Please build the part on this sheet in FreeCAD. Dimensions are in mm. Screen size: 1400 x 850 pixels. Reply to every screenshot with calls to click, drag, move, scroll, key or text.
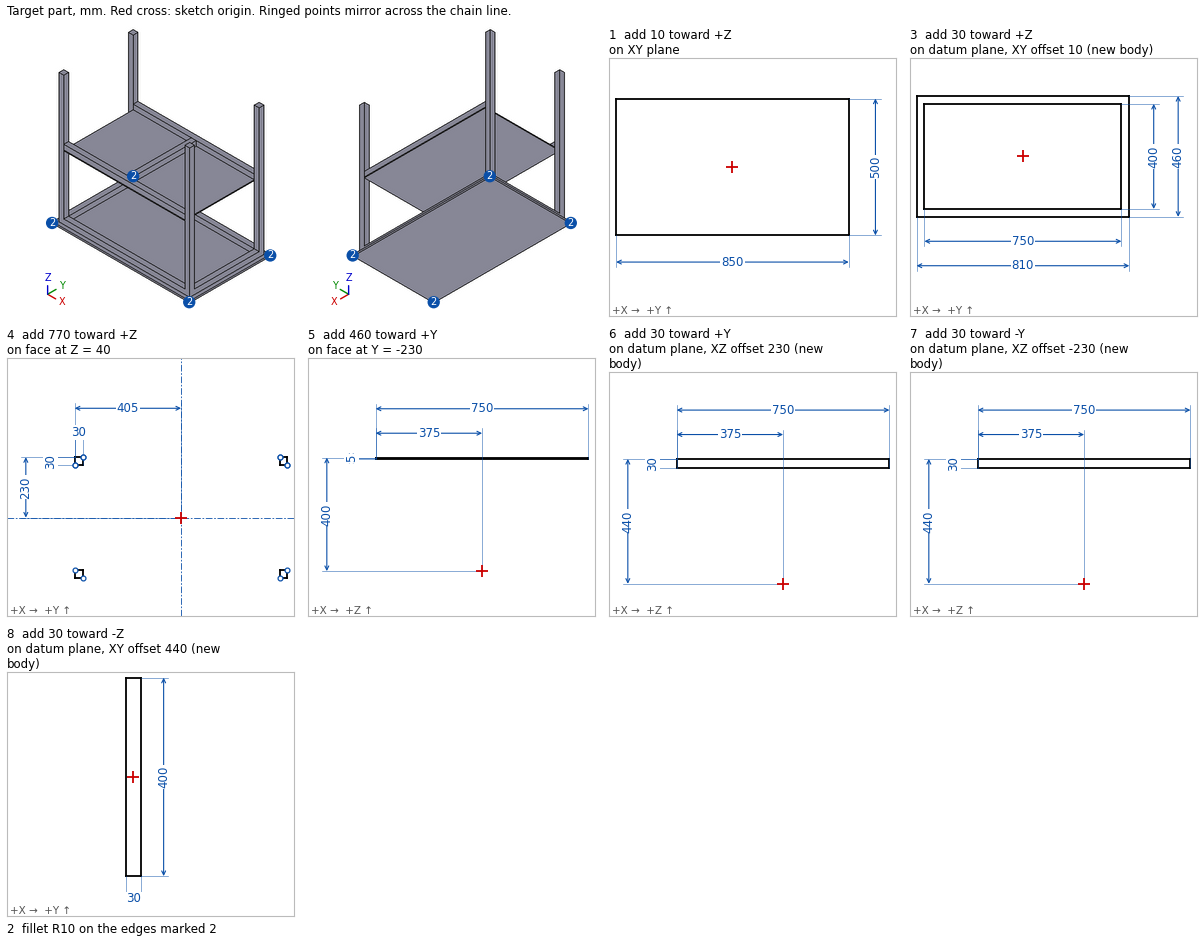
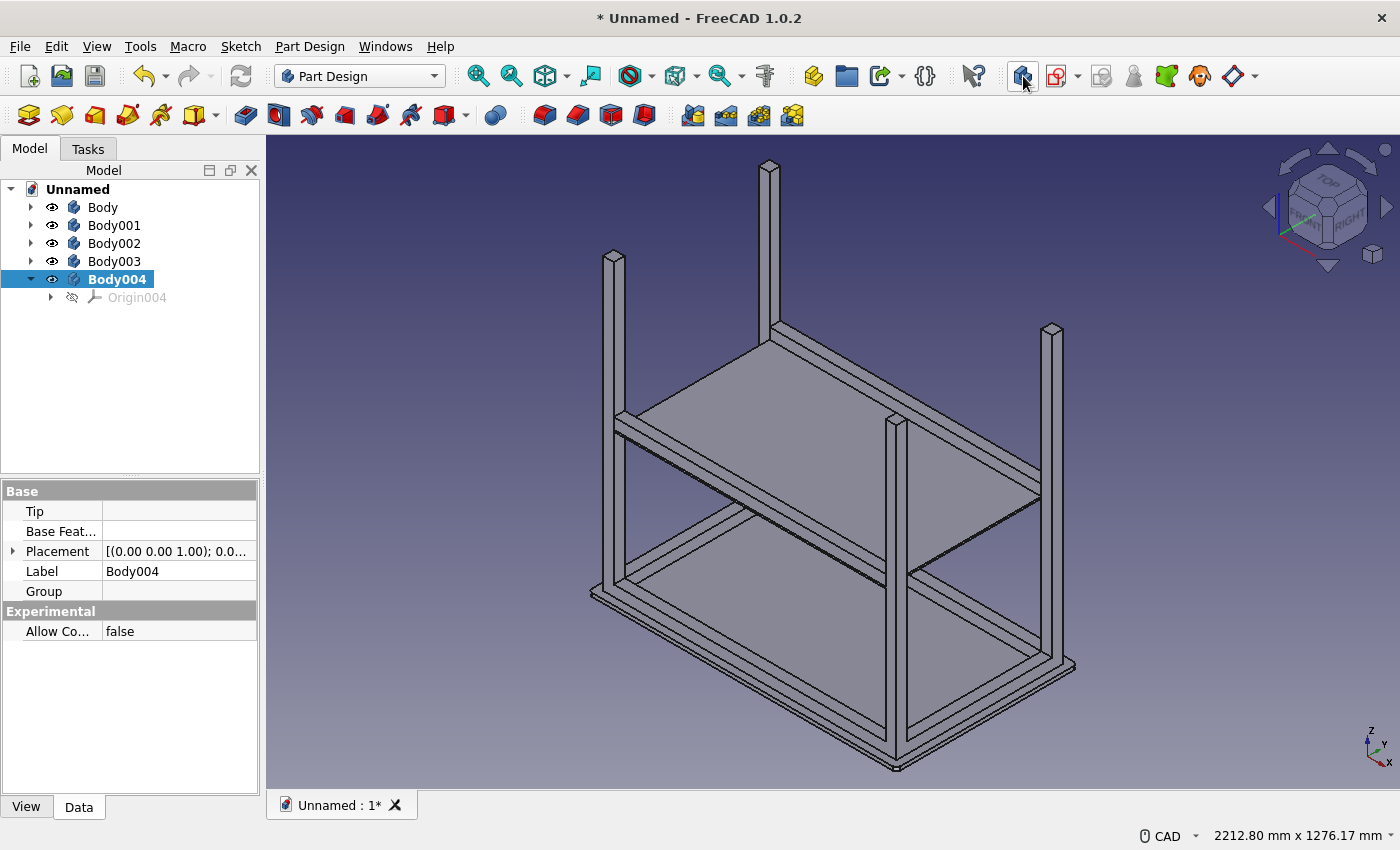
click(51, 297)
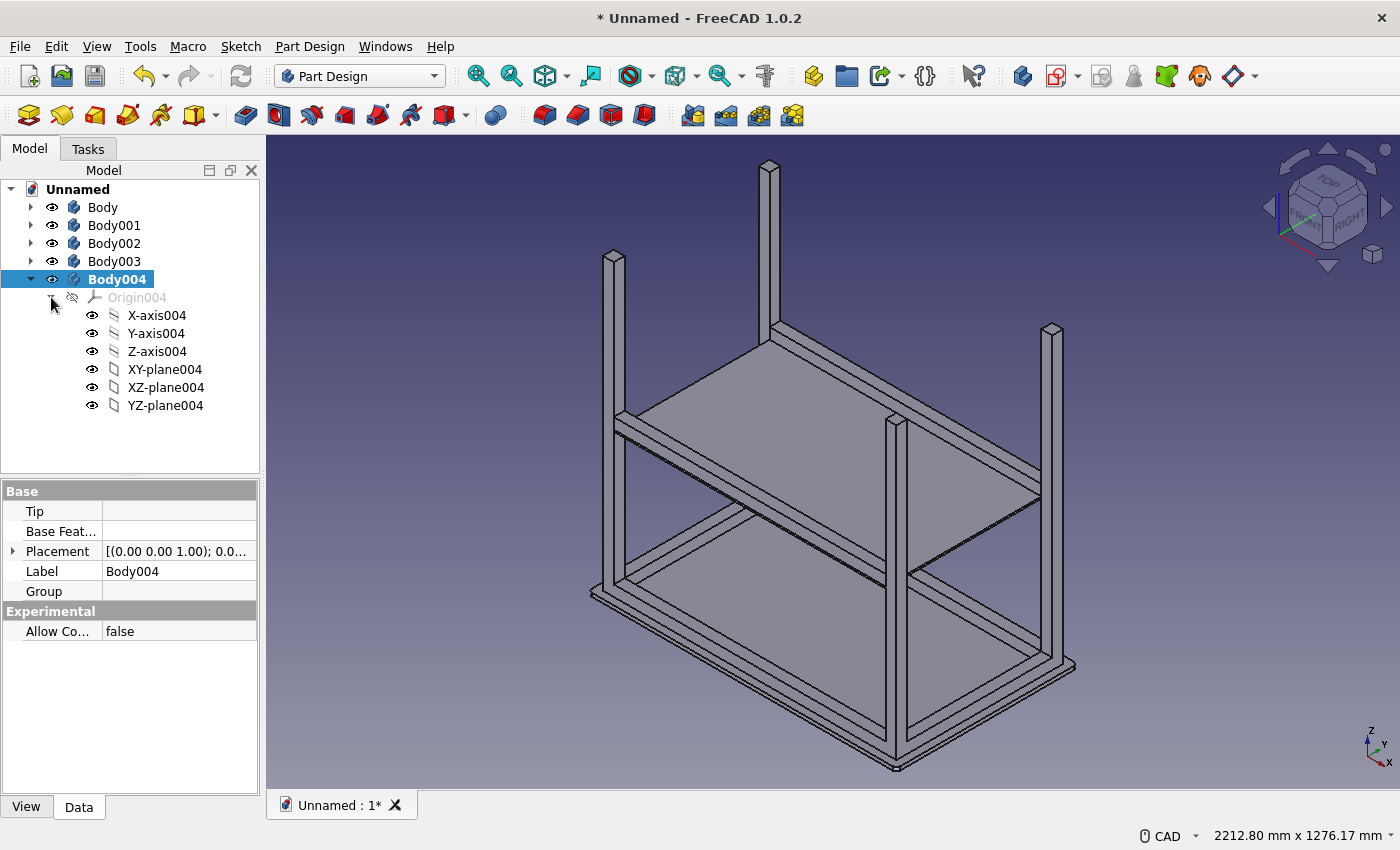
click(137, 369)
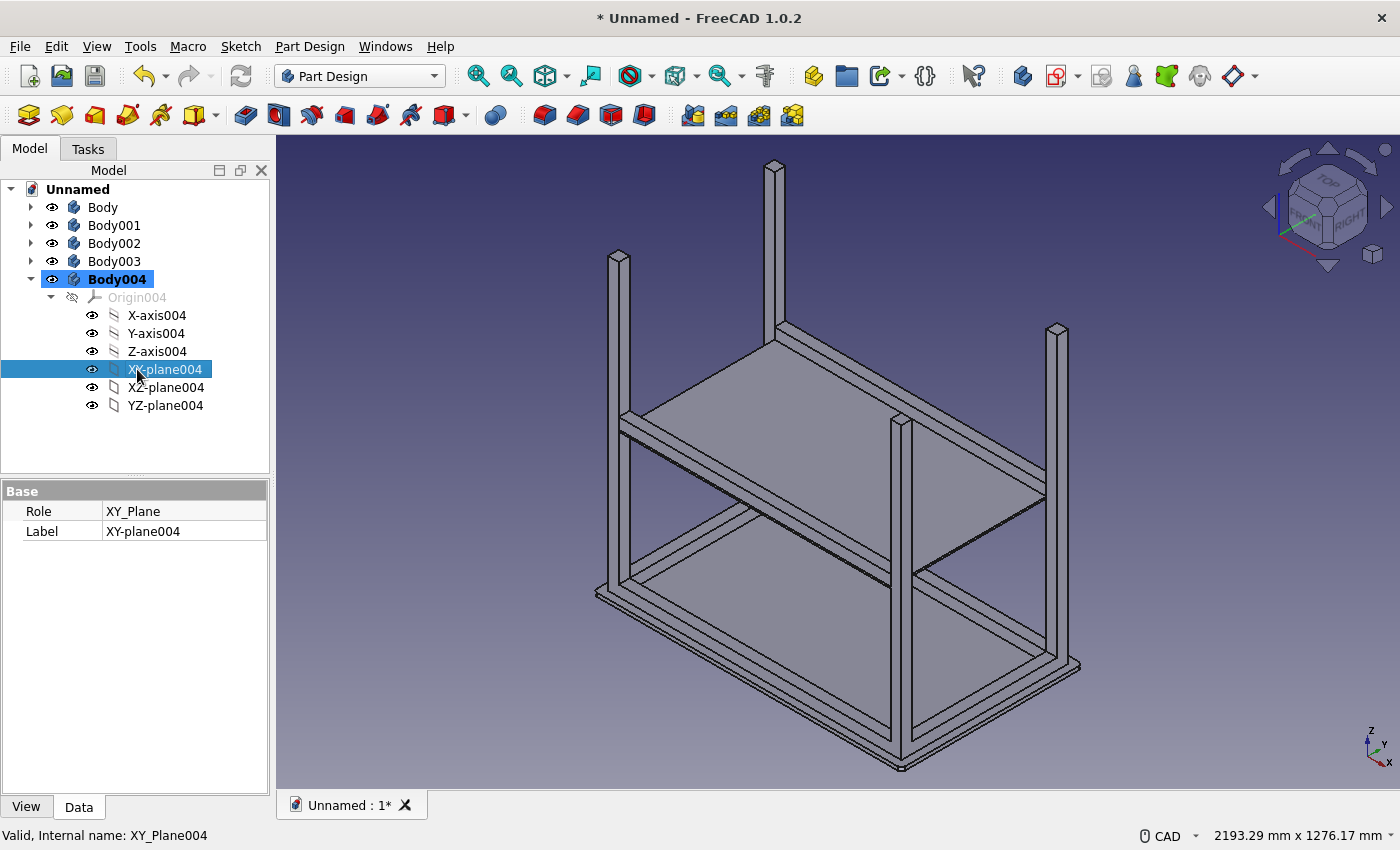
click(1232, 76)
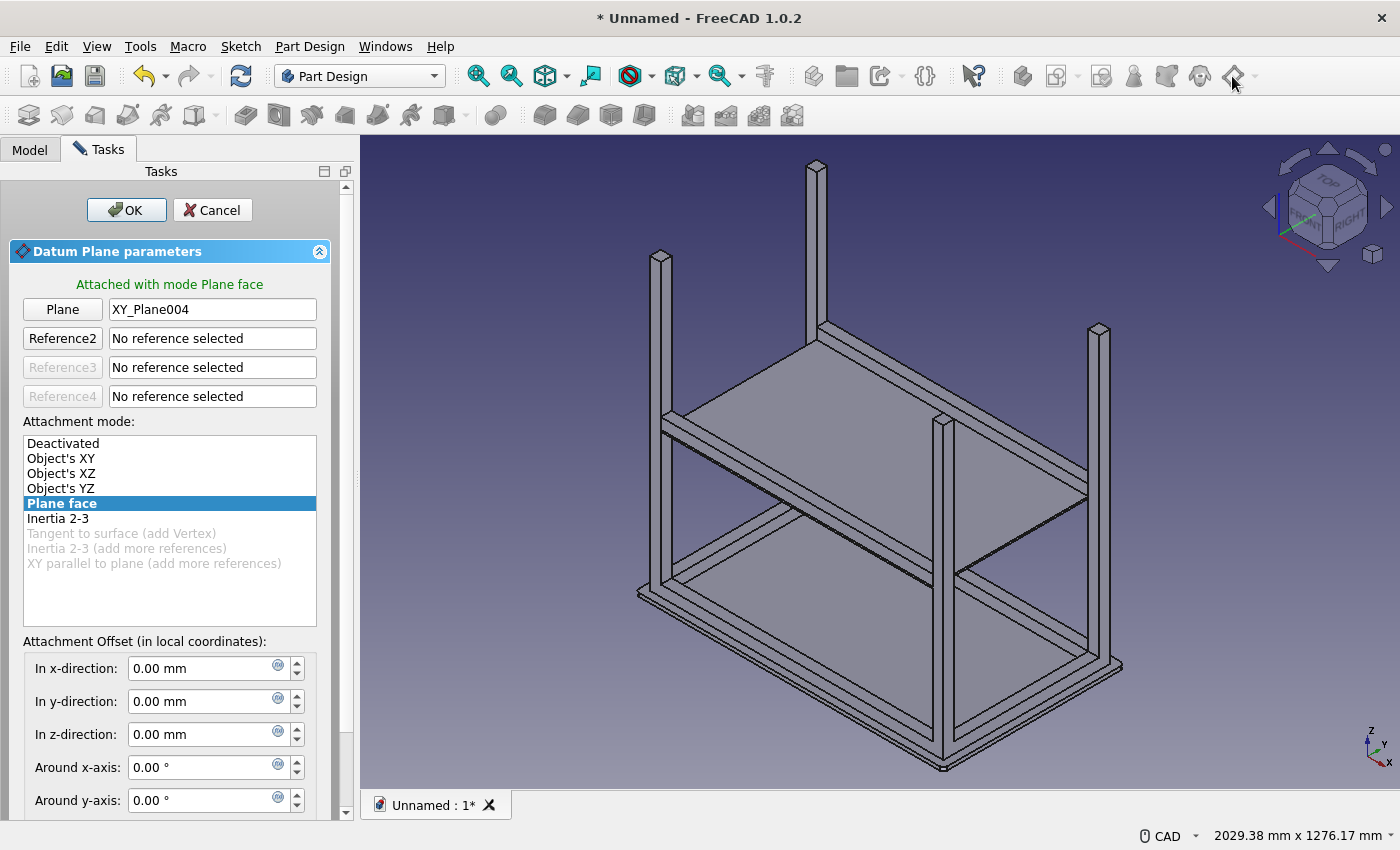
triple_click(210, 734)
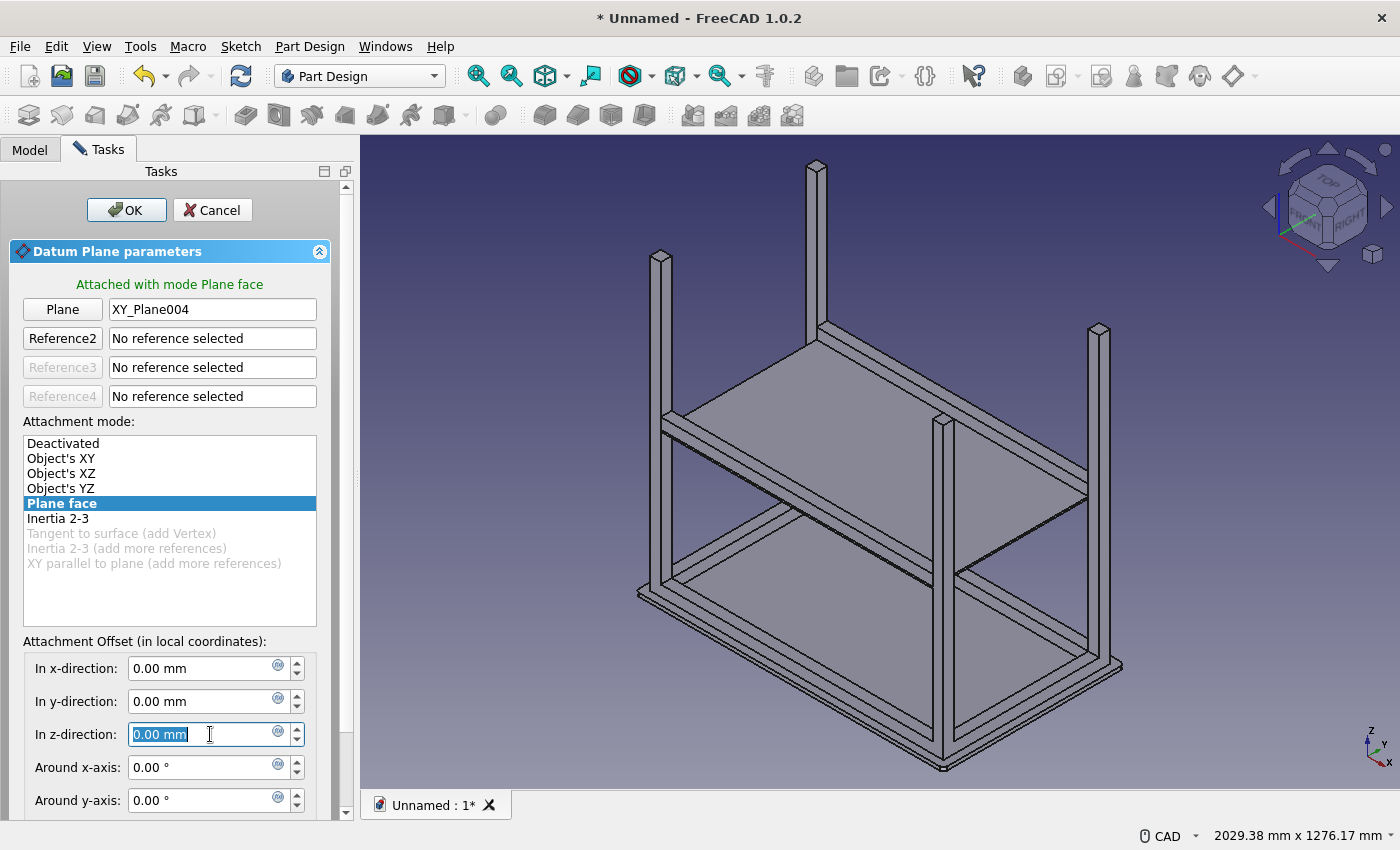
text(440)
key(Tab)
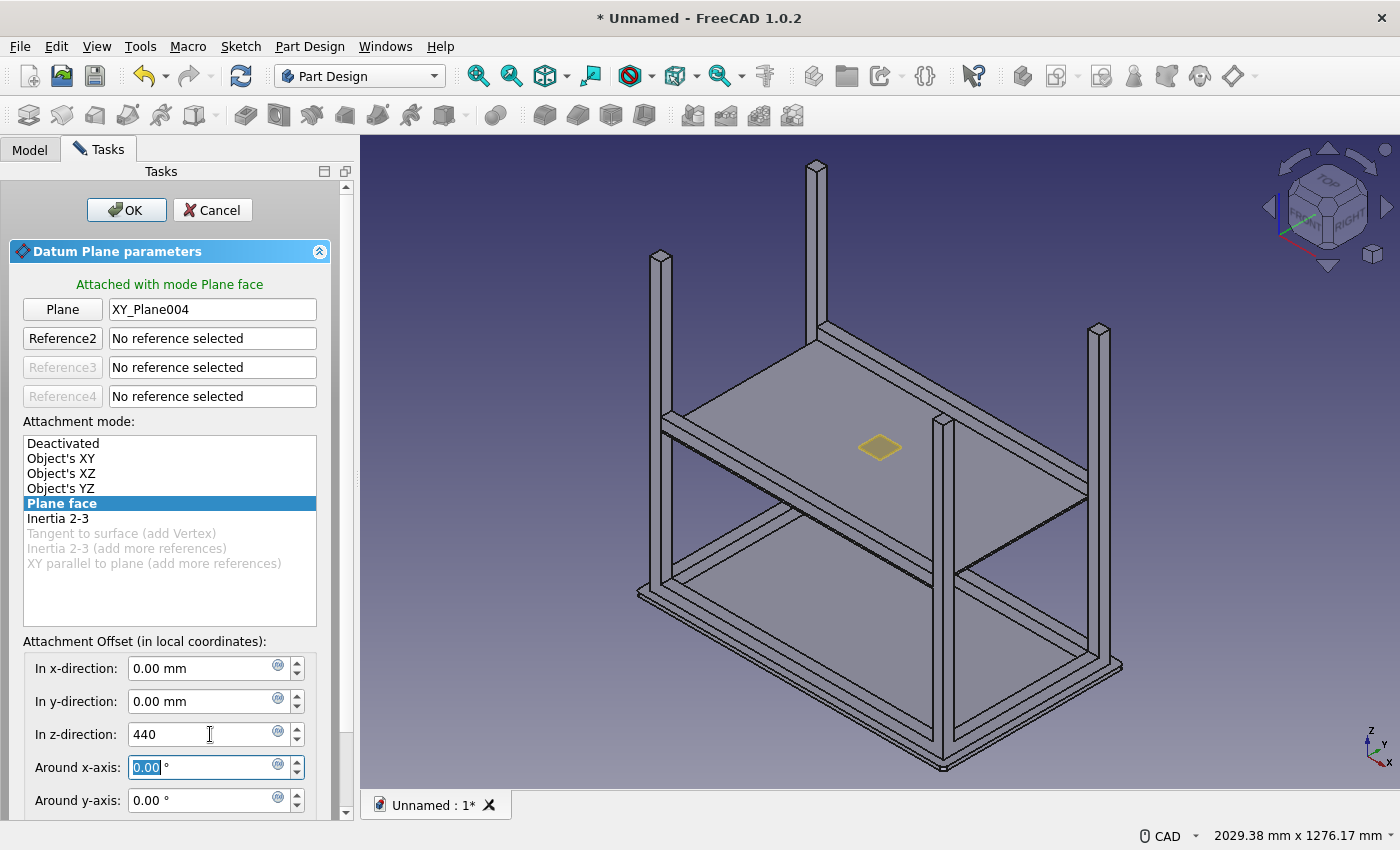
click(127, 210)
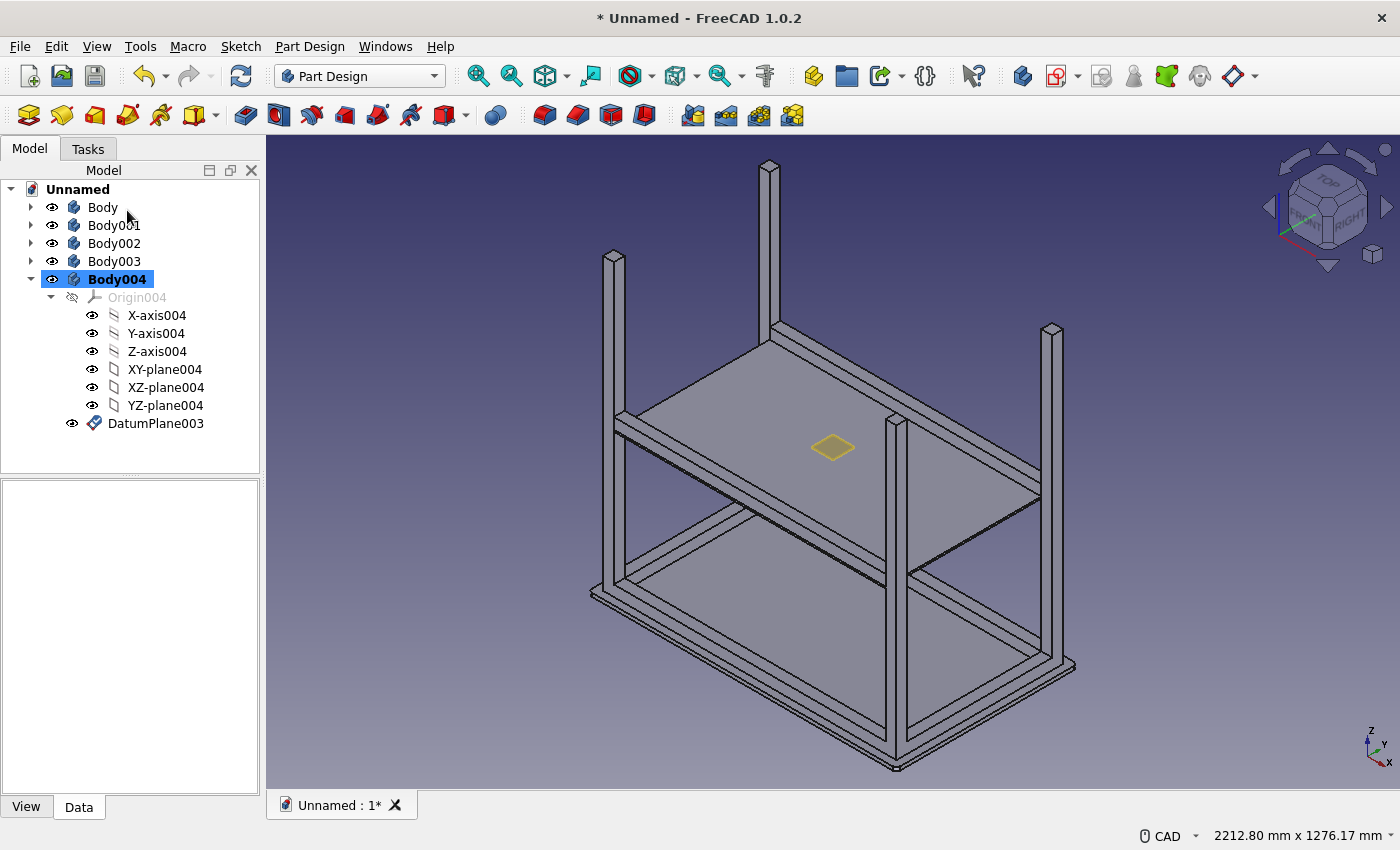
click(117, 423)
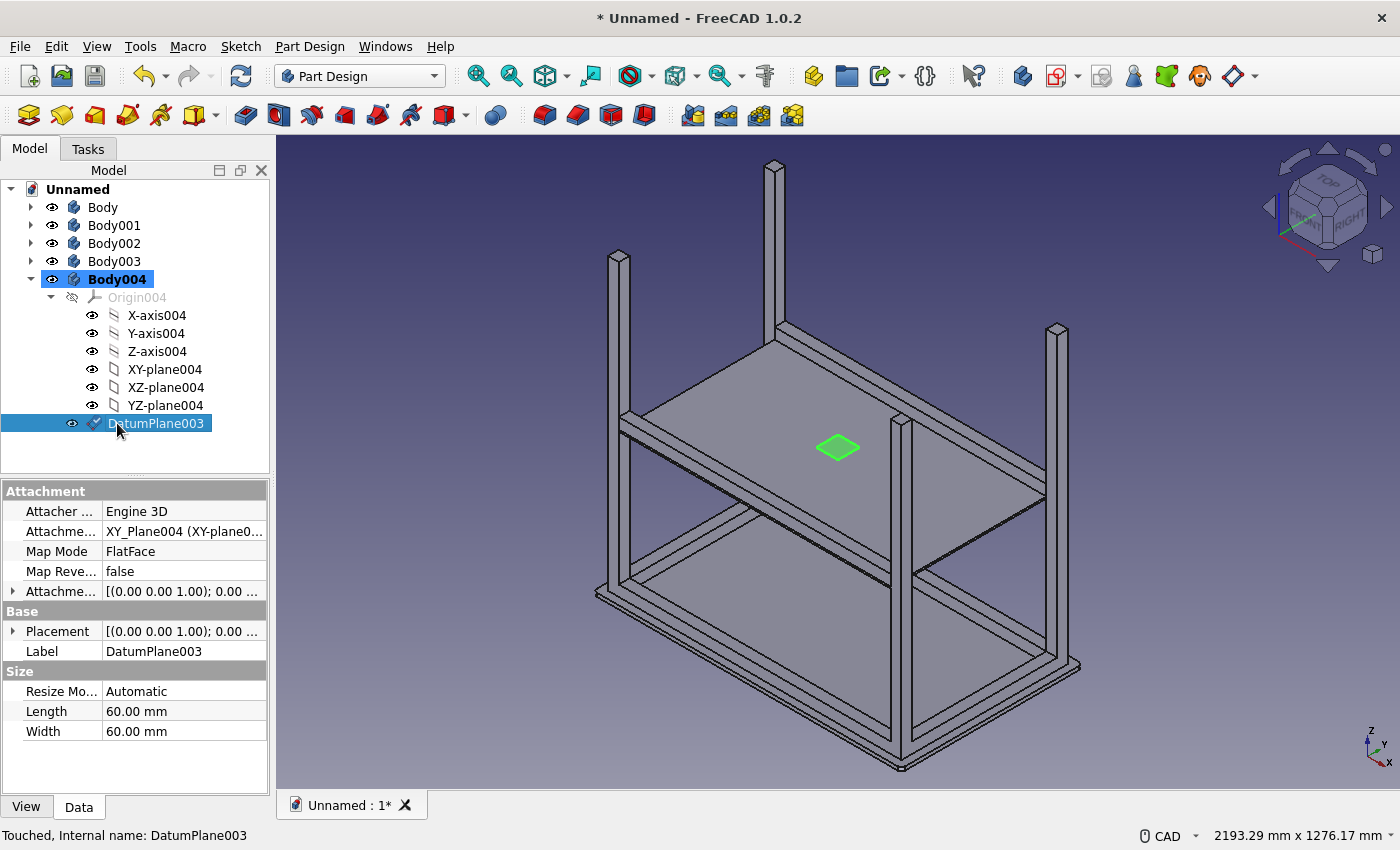
click(1056, 76)